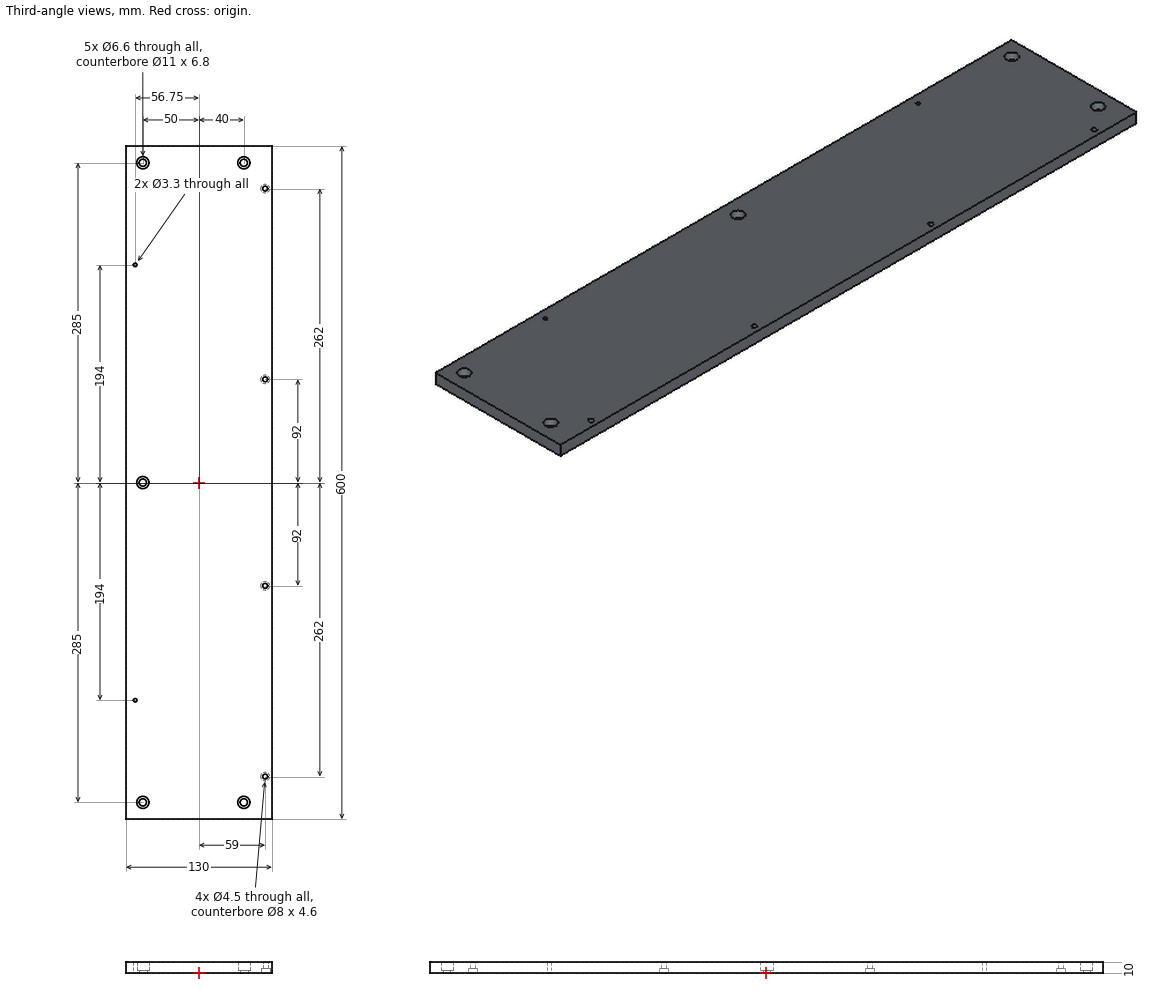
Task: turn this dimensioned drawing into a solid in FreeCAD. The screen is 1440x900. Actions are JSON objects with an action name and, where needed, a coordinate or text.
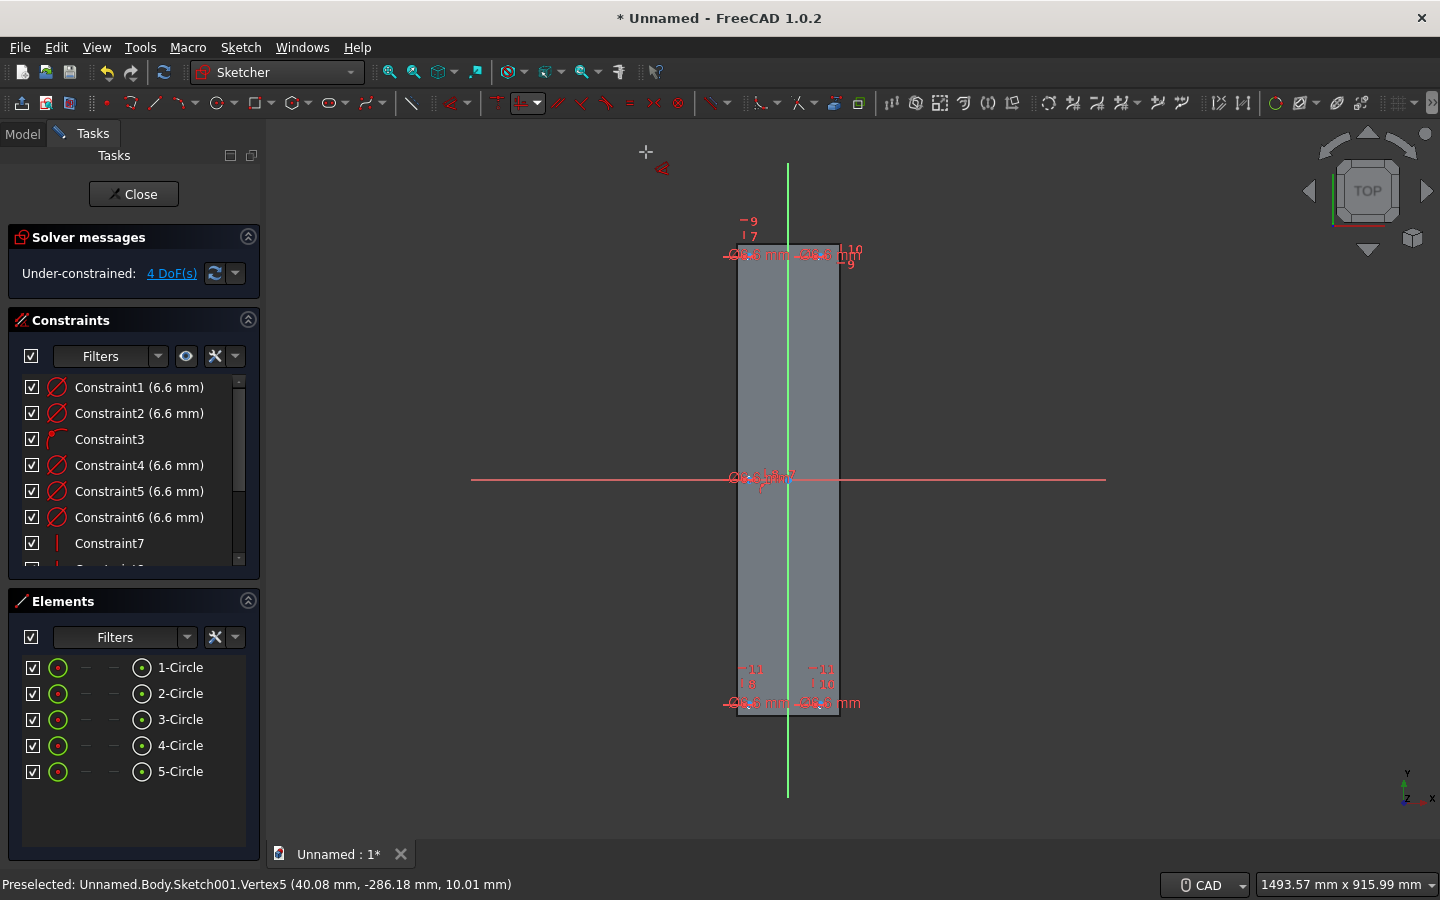
{"action": "left_click", "coordinate": [749, 257]}
{"action": "left_click", "coordinate": [769, 223]}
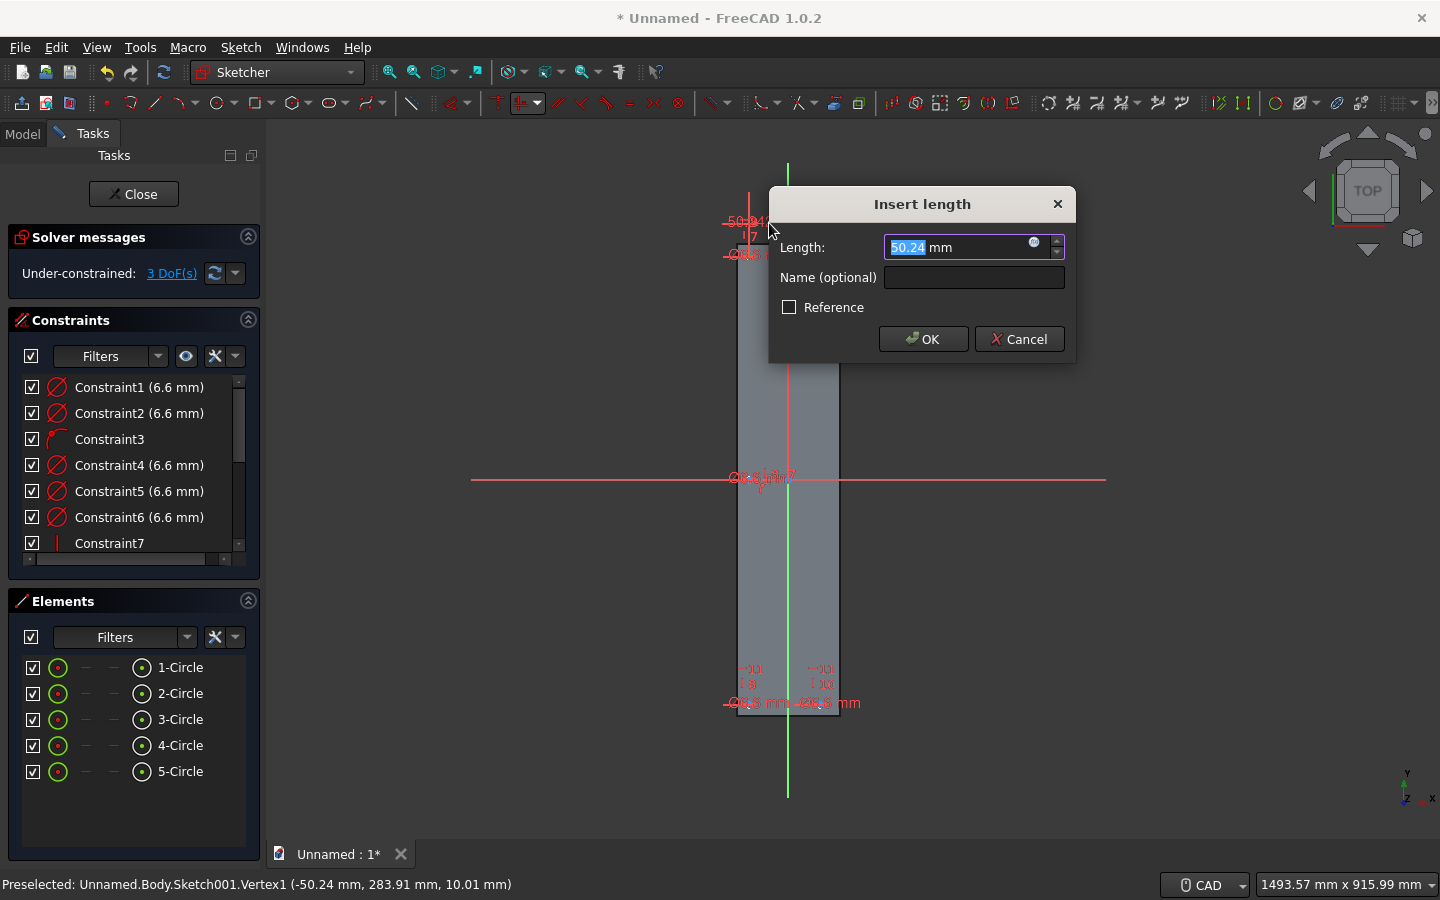
{"action": "type", "text": "50"}
{"action": "key", "text": "Return"}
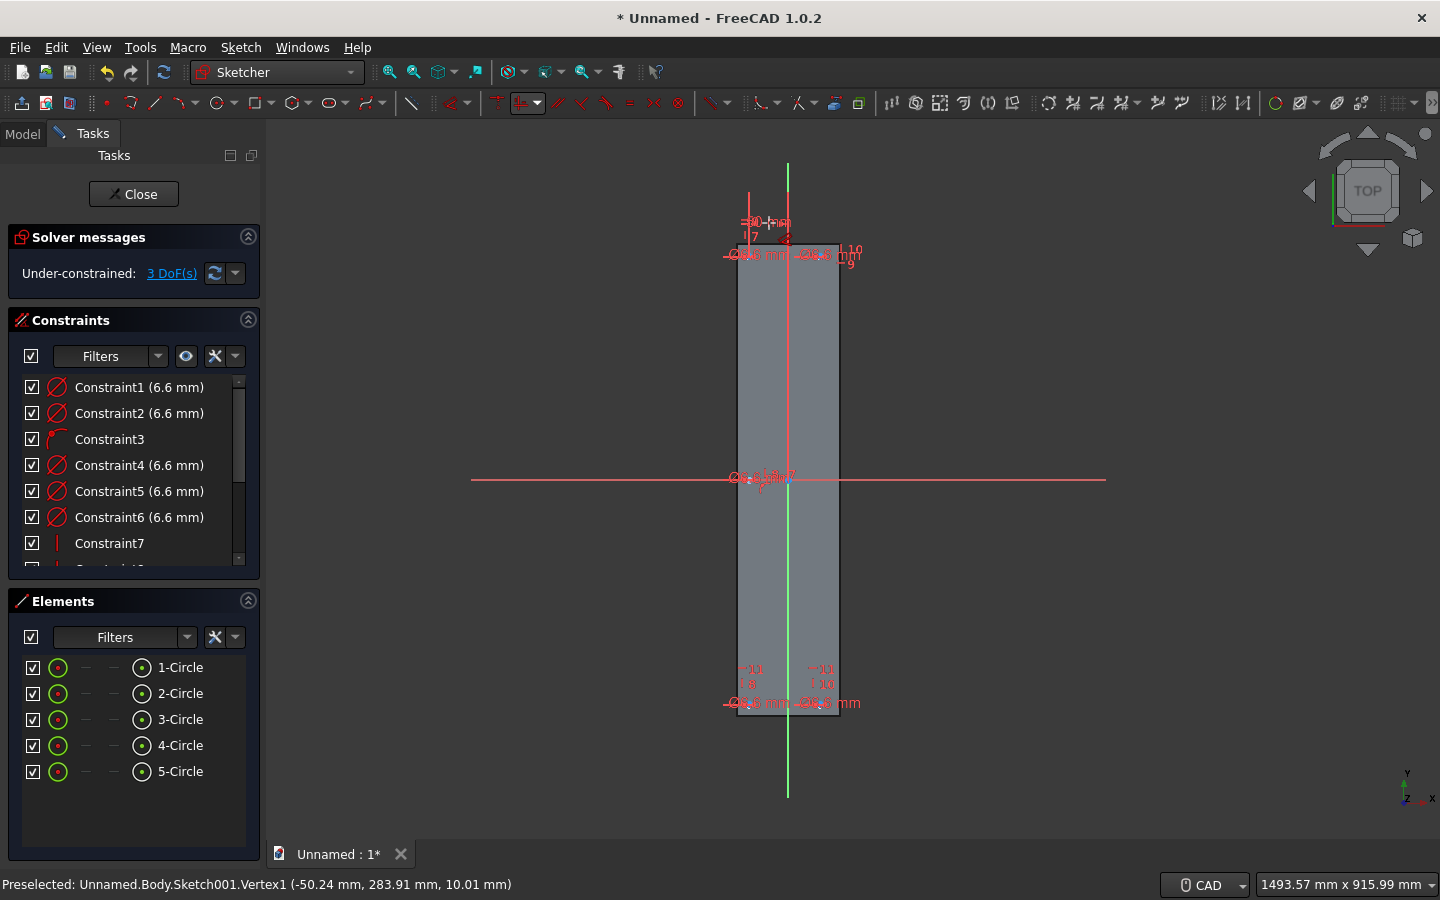
{"action": "scroll", "coordinate": [820, 257], "scroll_direction": "up", "scroll_amount": 2}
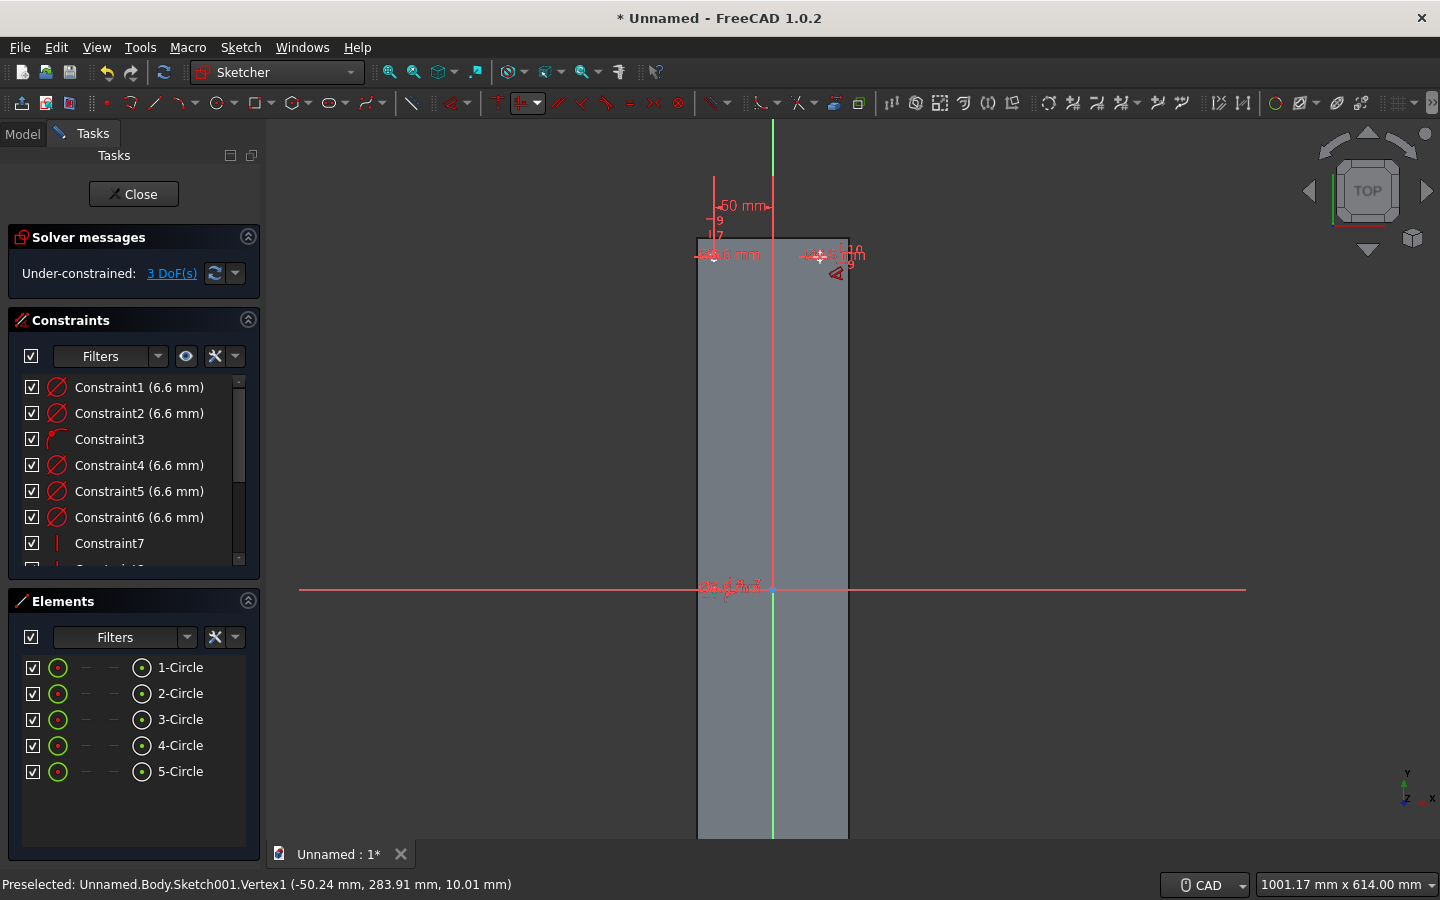
{"action": "left_click", "coordinate": [820, 257]}
{"action": "left_click", "coordinate": [796, 624]}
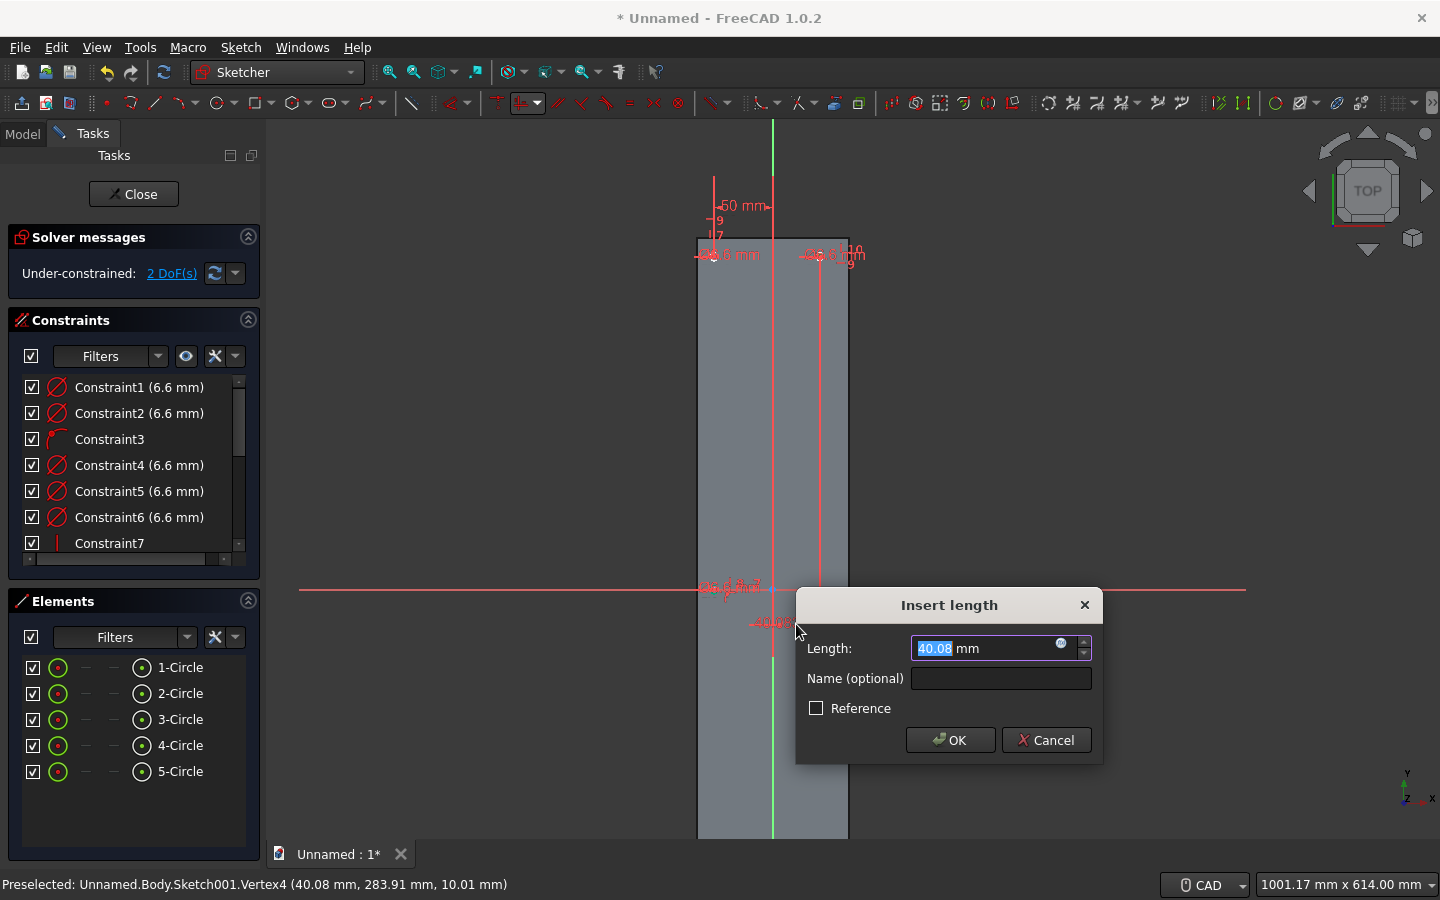
{"action": "type", "text": "40"}
{"action": "key", "text": "Return"}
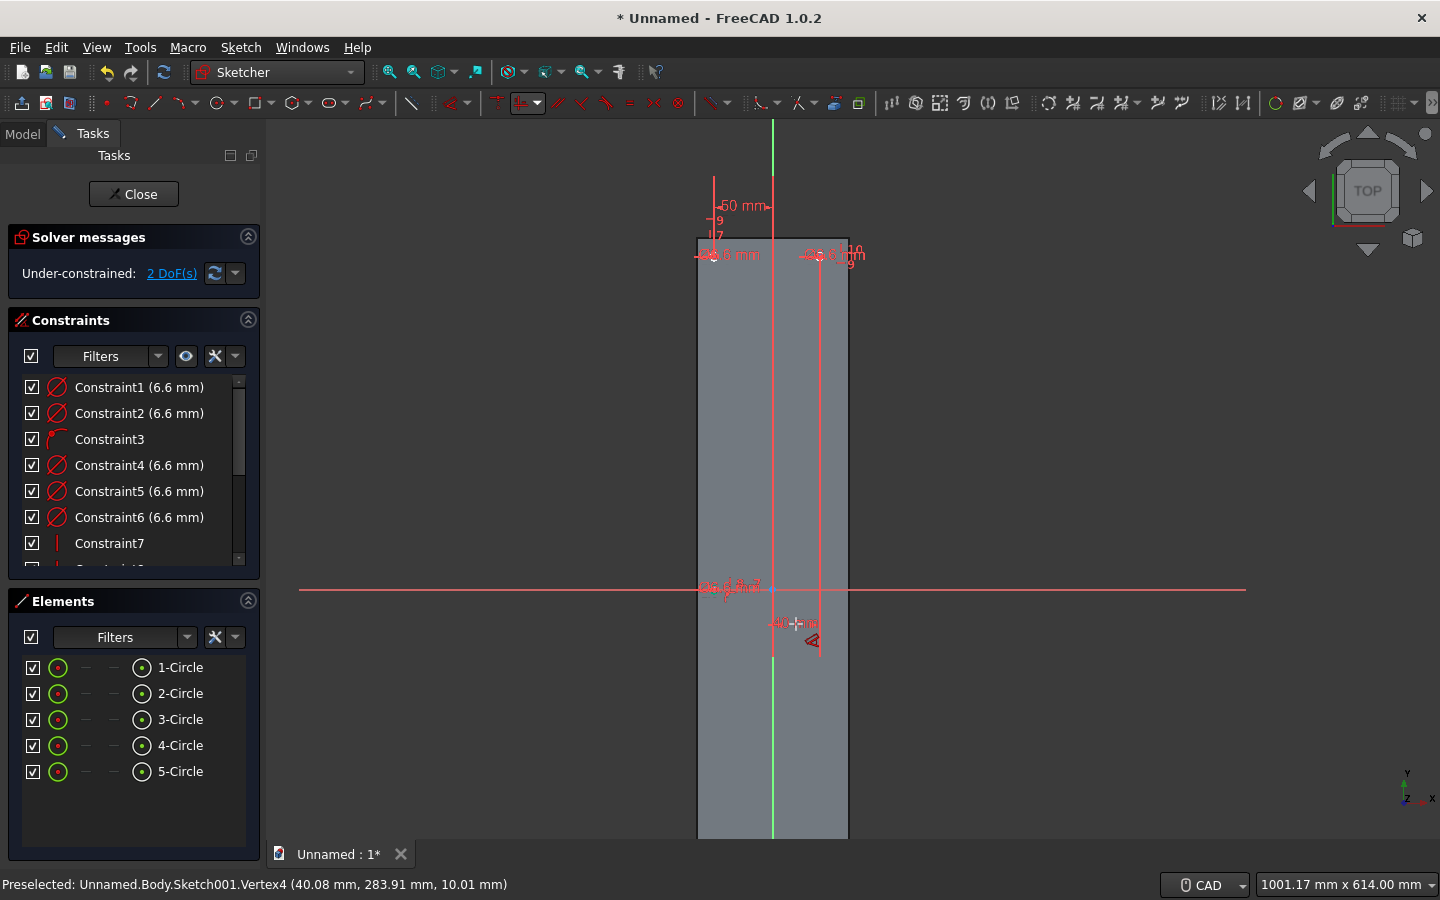
{"action": "left_click", "coordinate": [714, 257]}
{"action": "left_click", "coordinate": [680, 423]}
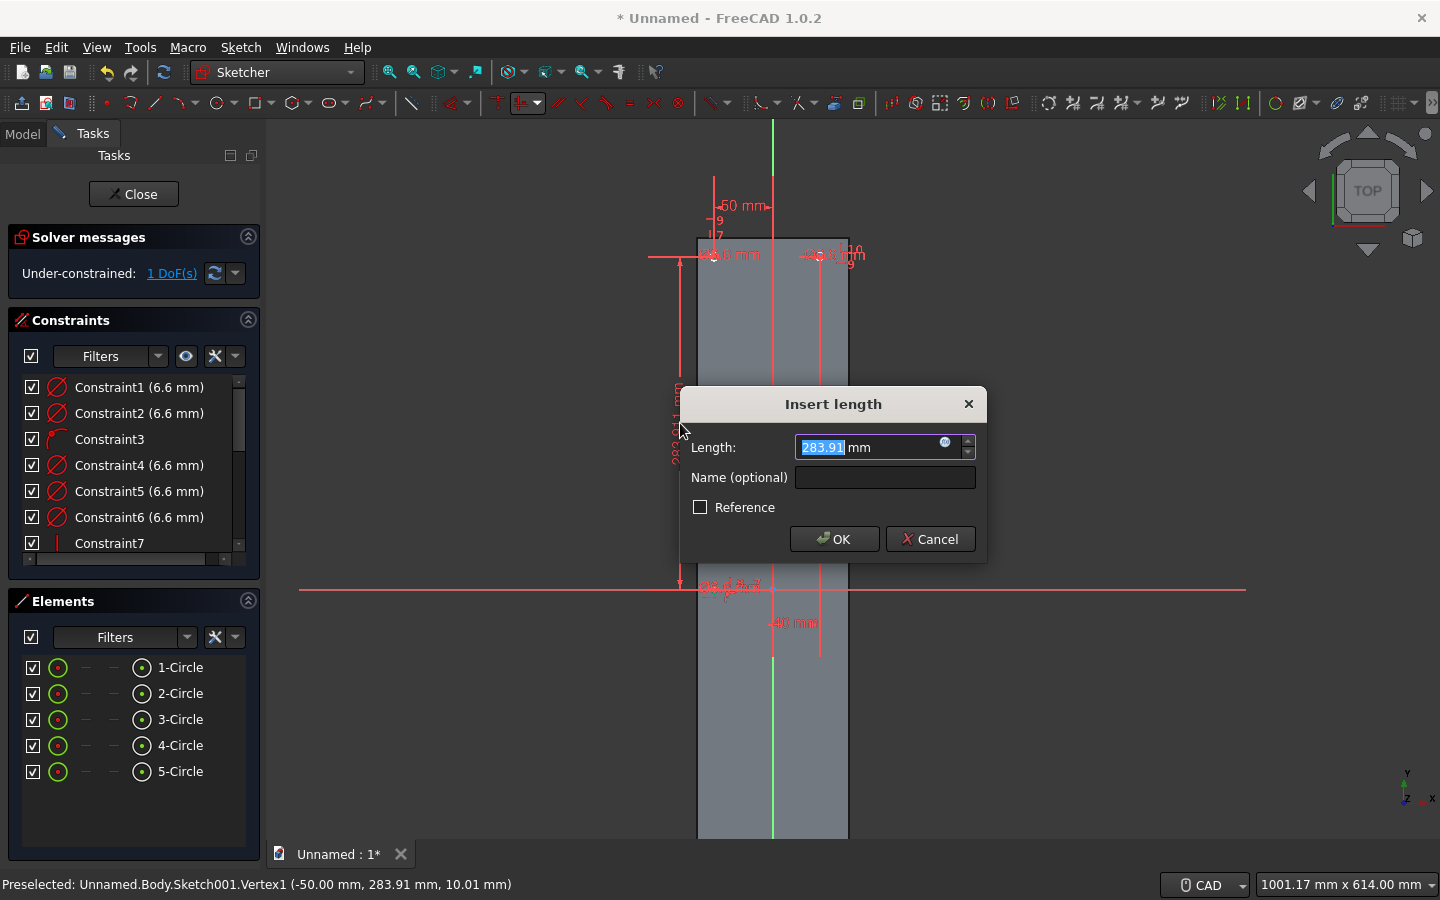
{"action": "type", "text": "285"}
{"action": "key", "text": "Return"}